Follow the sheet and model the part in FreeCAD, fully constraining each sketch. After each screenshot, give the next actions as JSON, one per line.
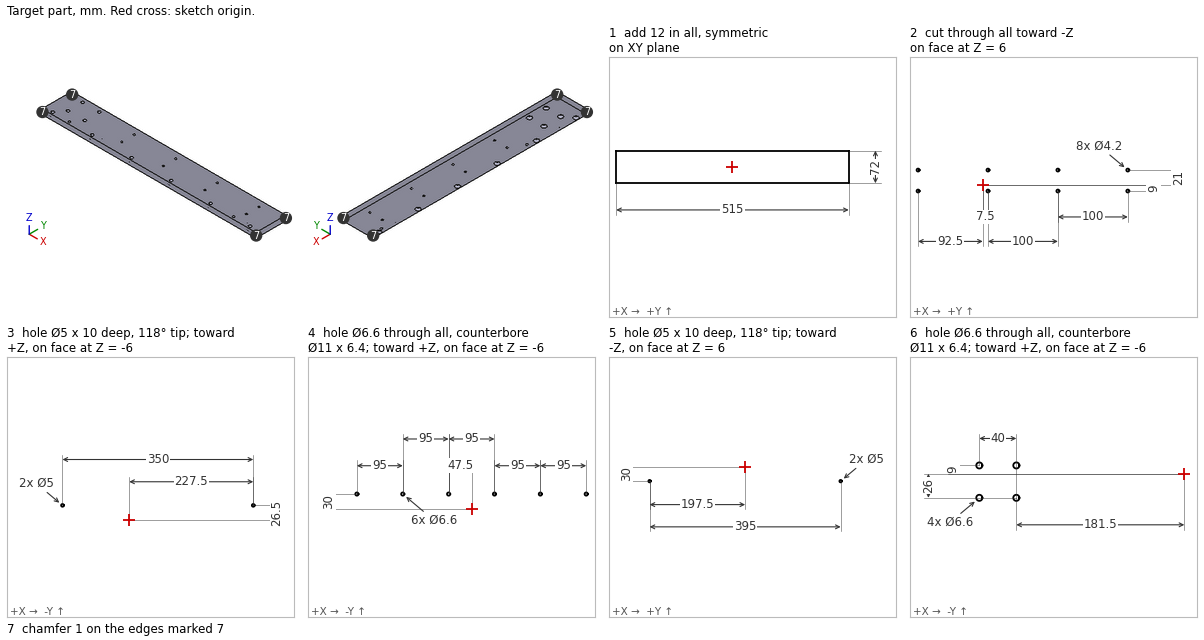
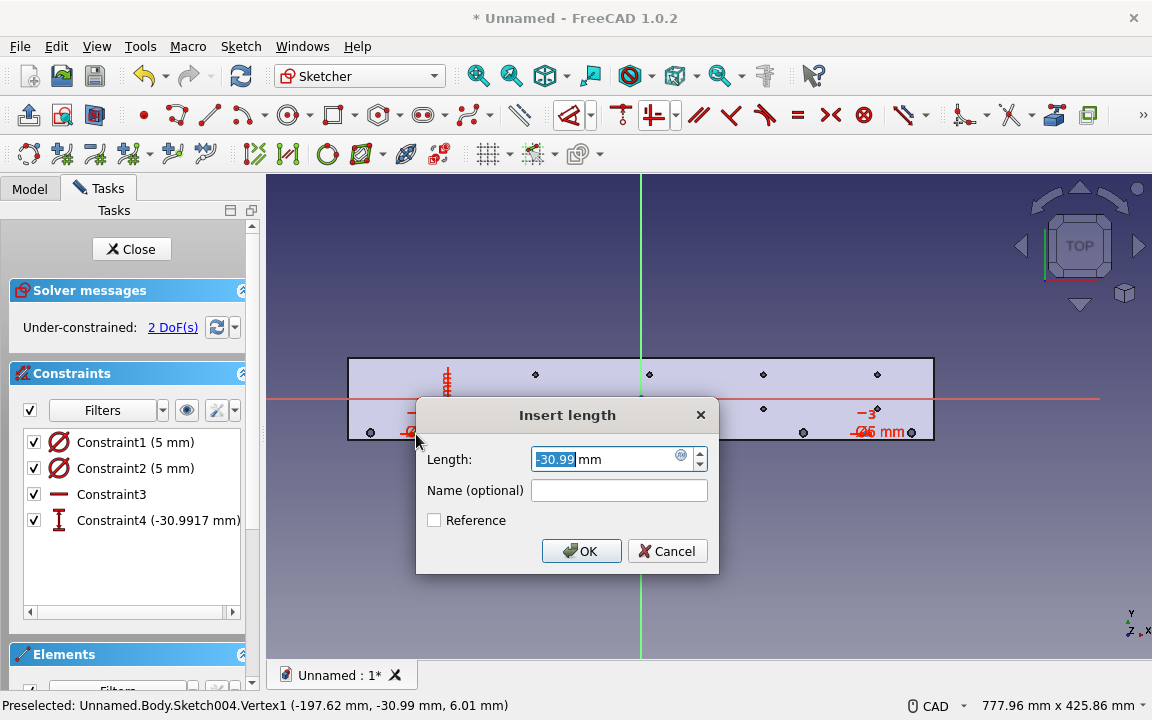
{"action": "type", "text": "-30"}
{"action": "key", "text": "Return"}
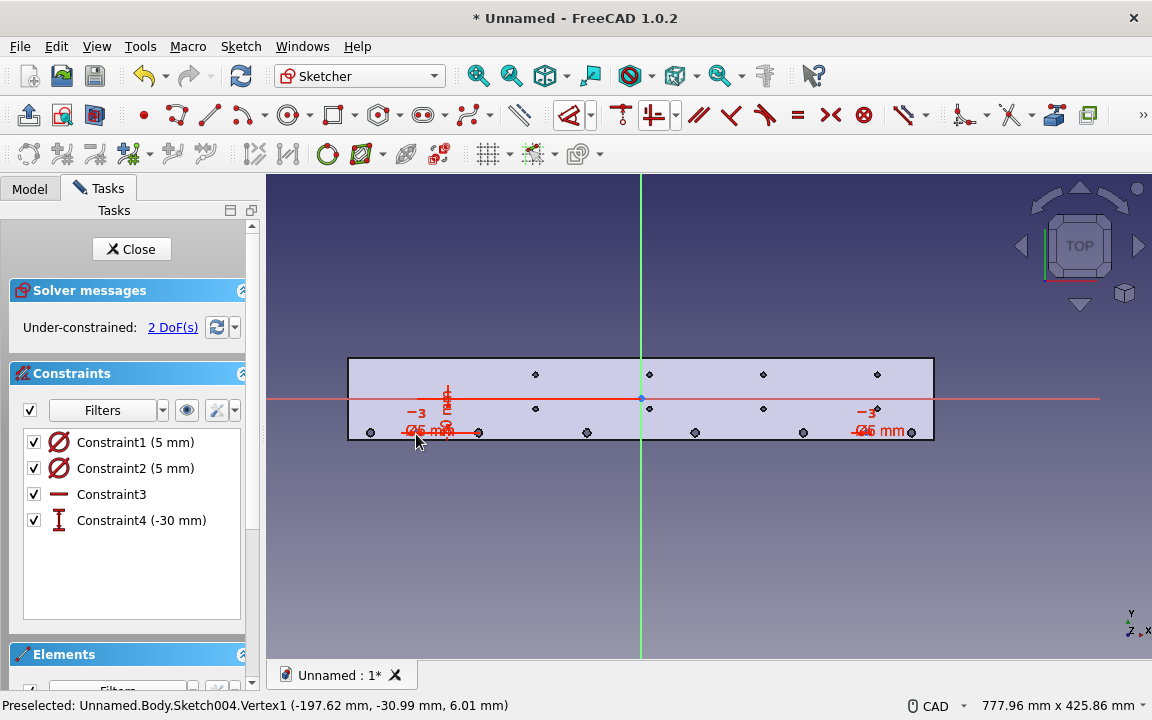
{"action": "left_click", "coordinate": [416, 433]}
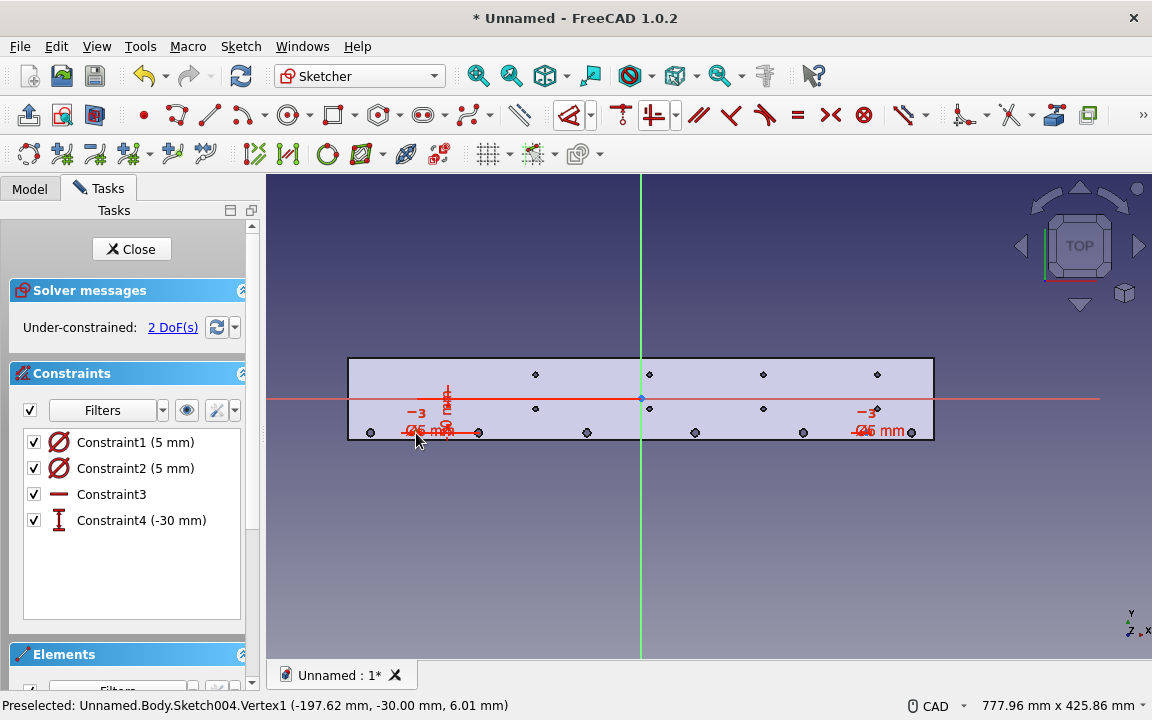
{"action": "left_click", "coordinate": [866, 433]}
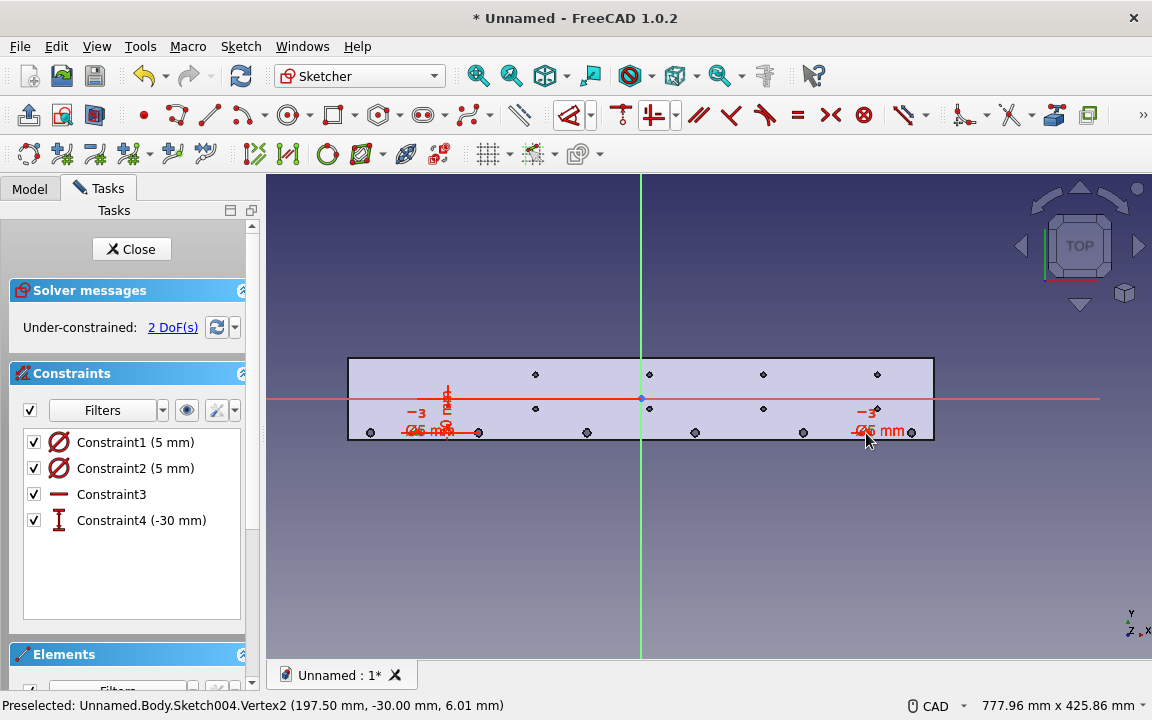
{"action": "key", "text": "l"}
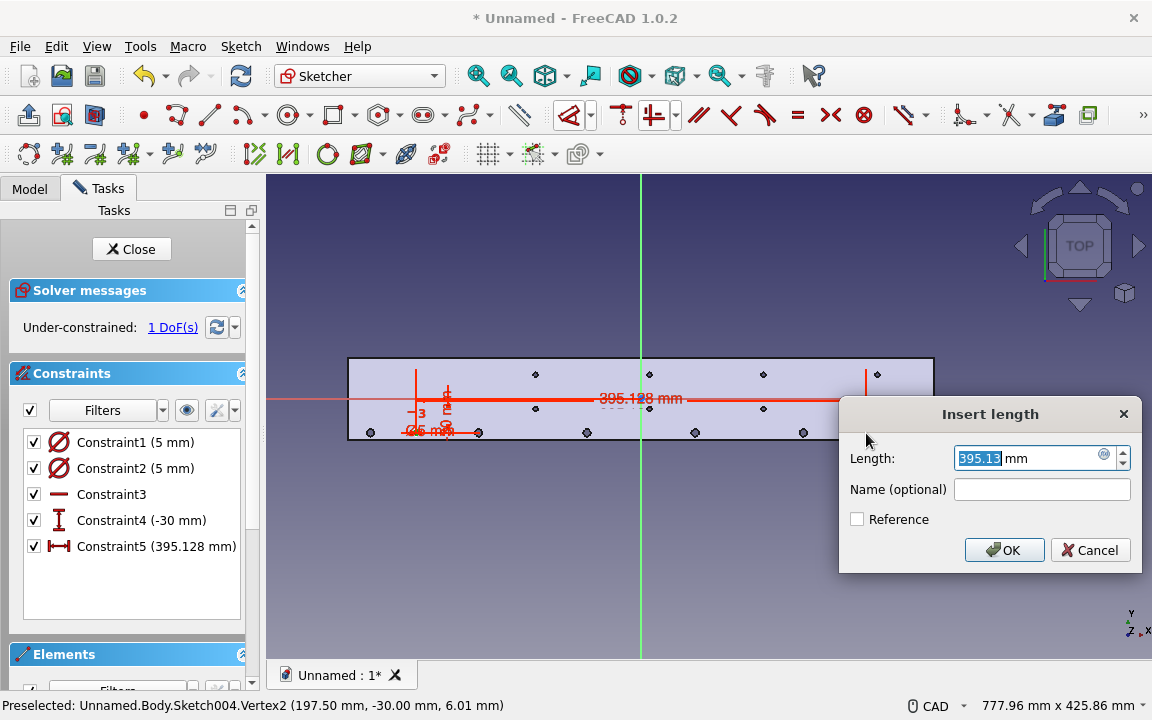
{"action": "type", "text": "395"}
{"action": "key", "text": "Return"}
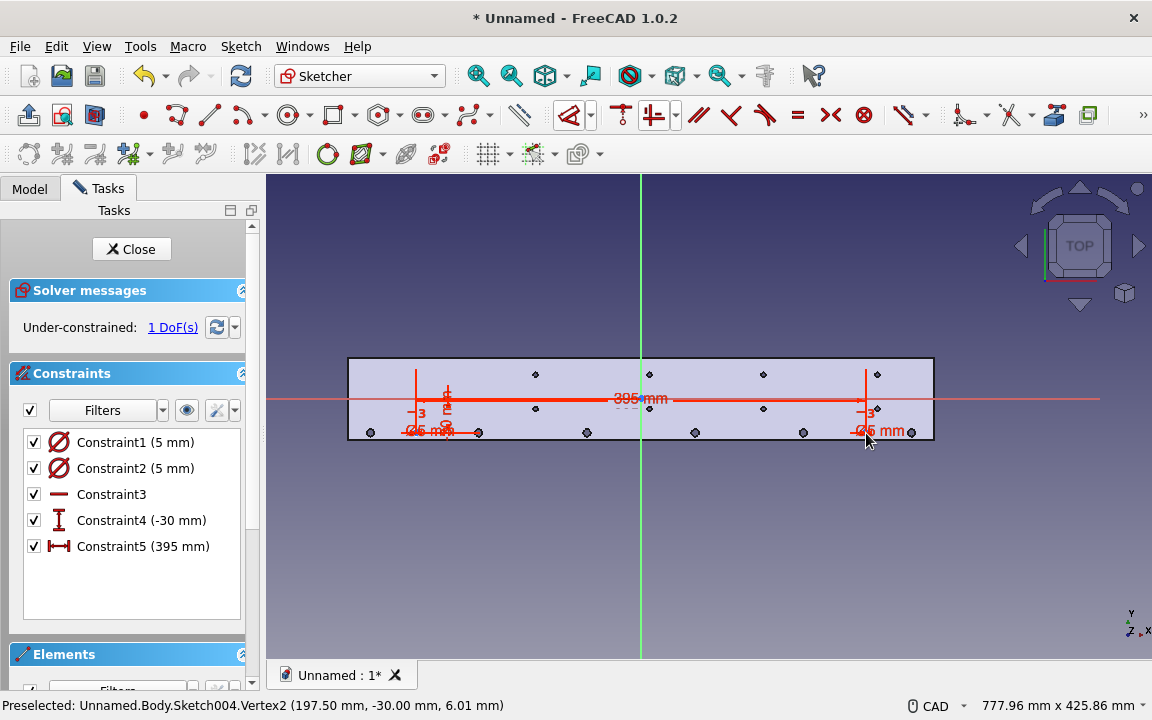
{"action": "left_click", "coordinate": [416, 433]}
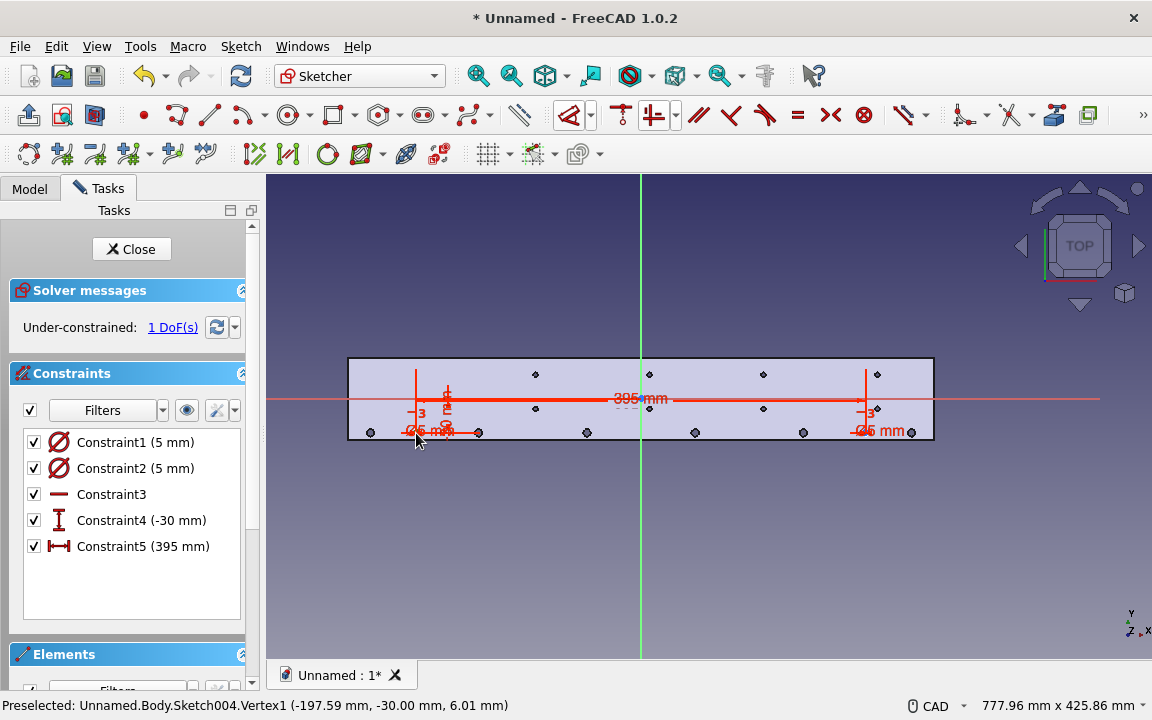
{"action": "left_click", "coordinate": [590, 116]}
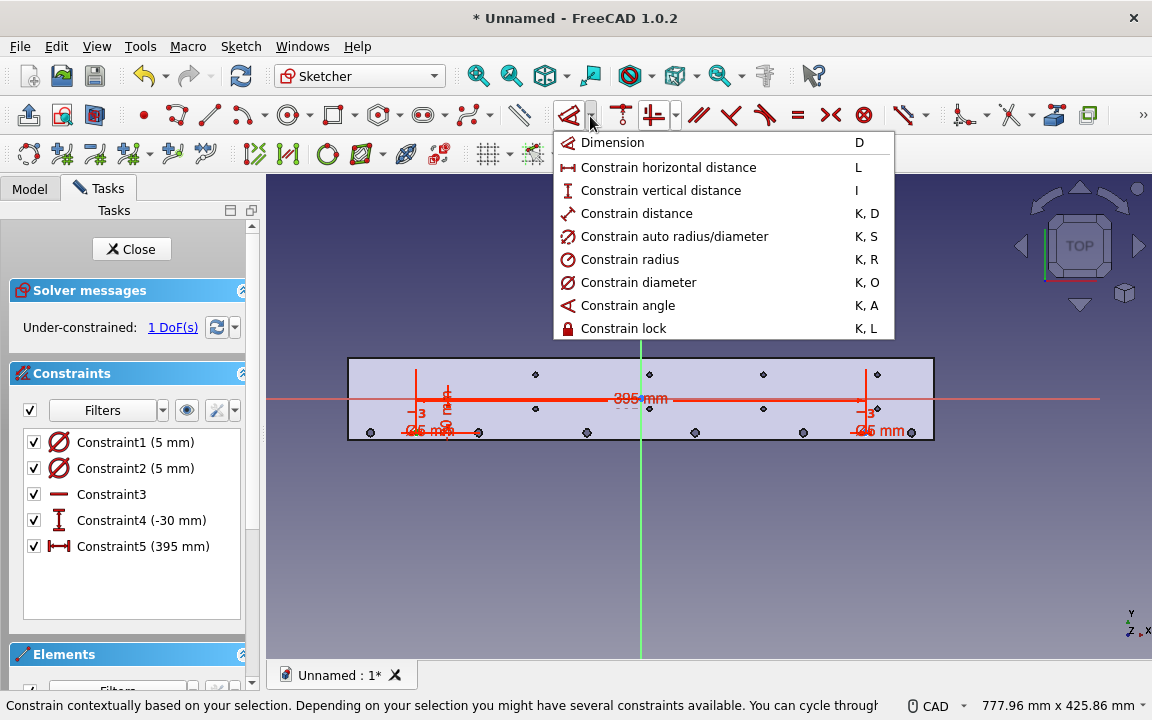
{"action": "left_click", "coordinate": [724, 168]}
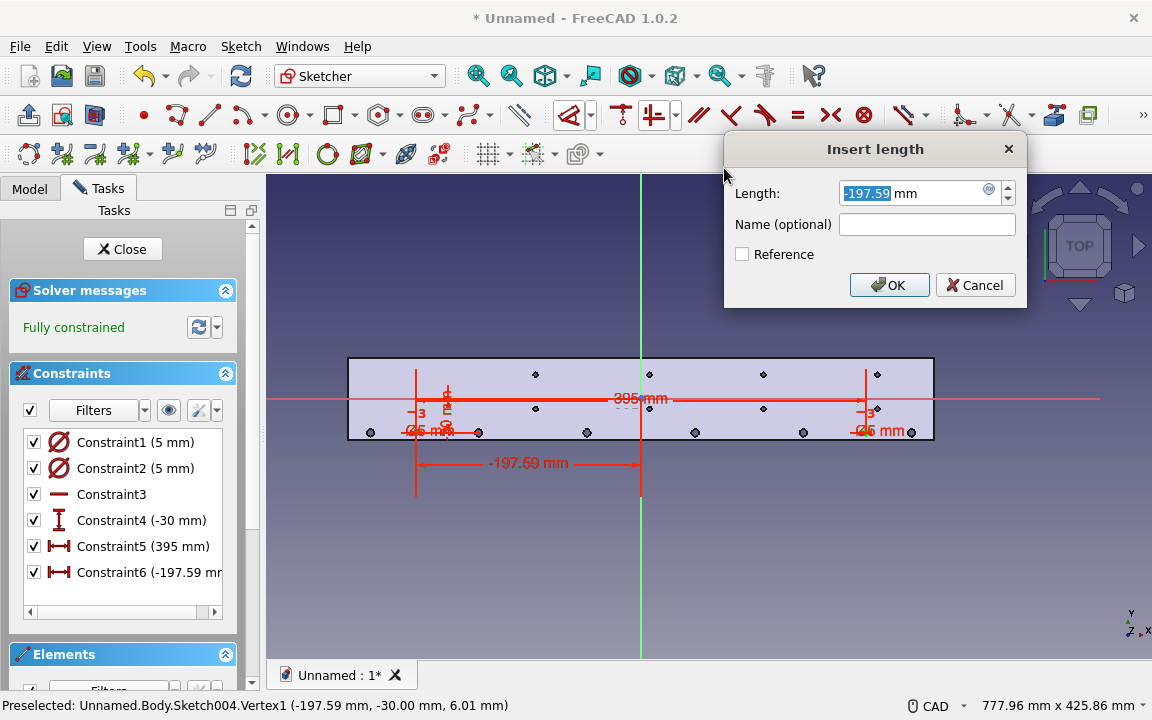
{"action": "type", "text": "-197.5"}
{"action": "key", "text": "Return"}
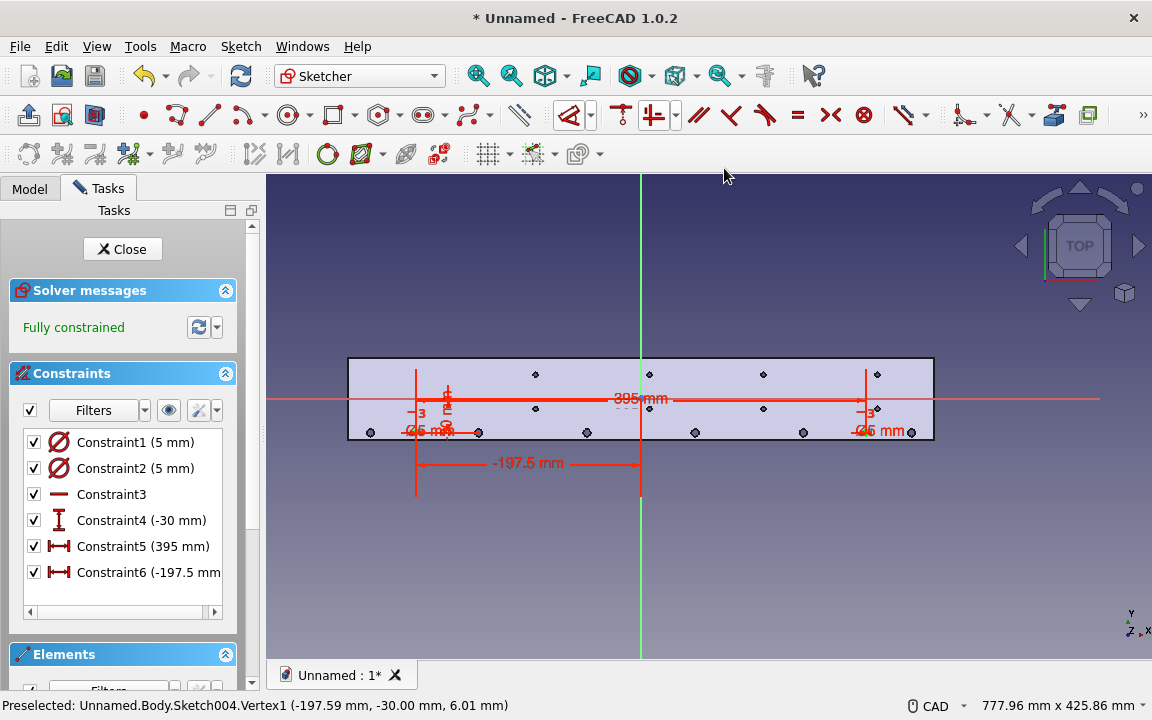
{"action": "left_click", "coordinate": [123, 249]}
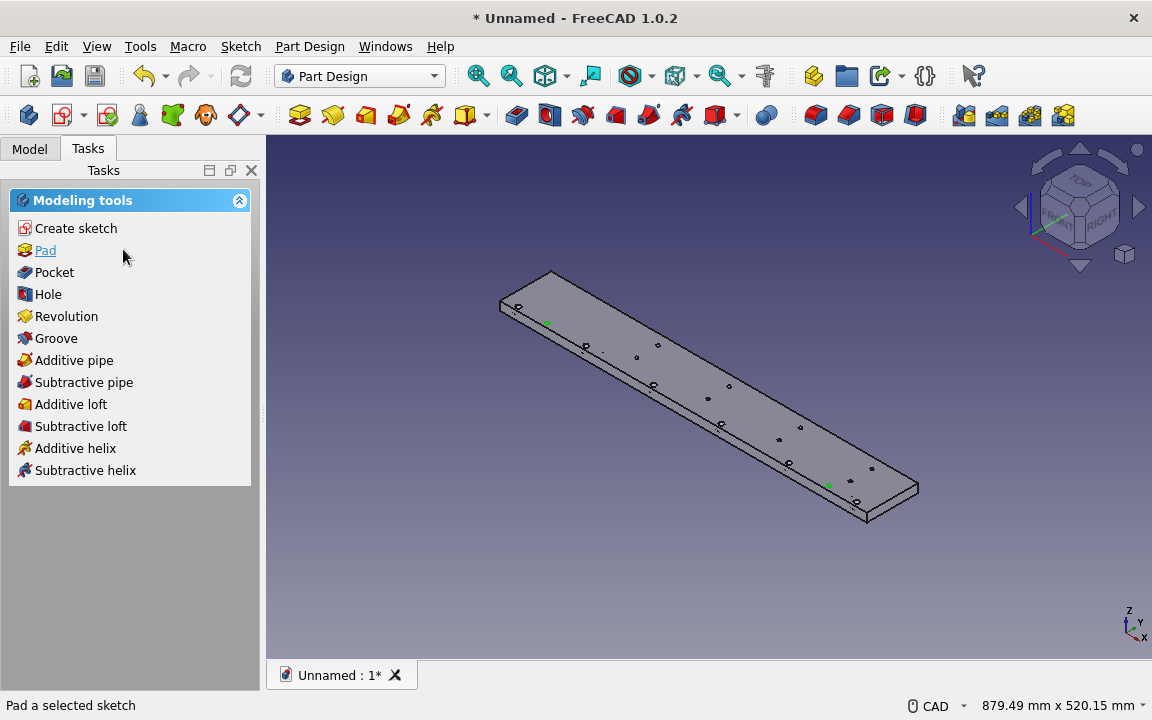
{"action": "left_click", "coordinate": [550, 116]}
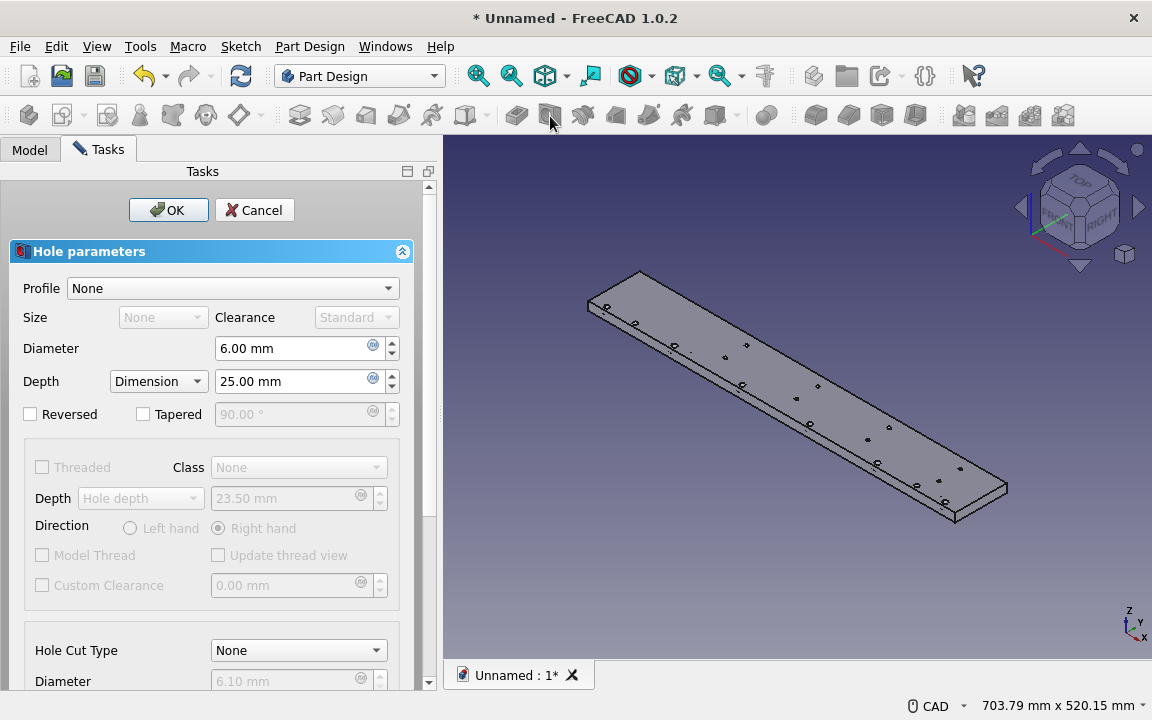
{"action": "triple_click", "coordinate": [300, 348]}